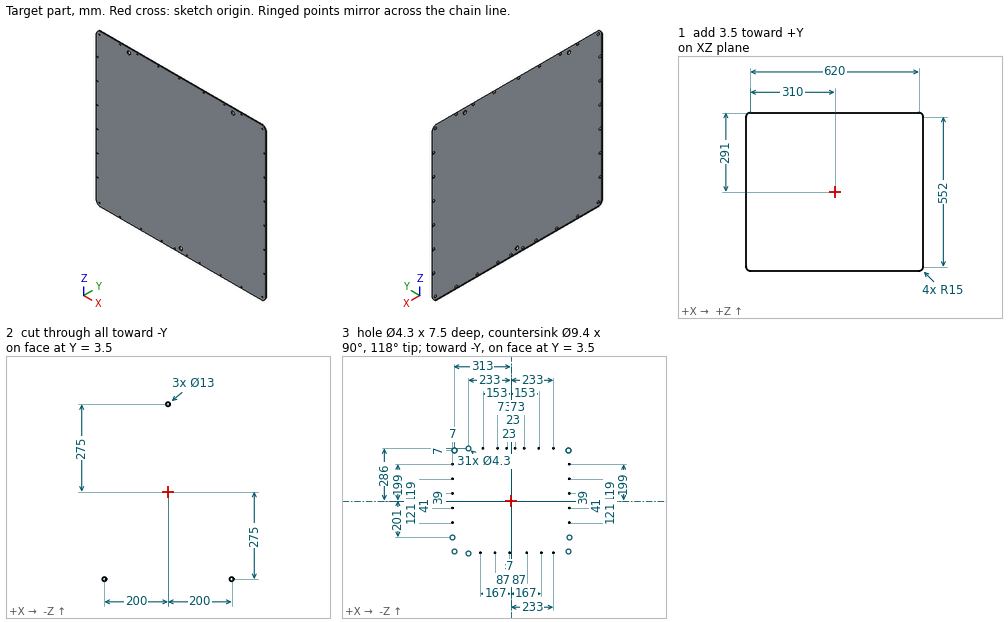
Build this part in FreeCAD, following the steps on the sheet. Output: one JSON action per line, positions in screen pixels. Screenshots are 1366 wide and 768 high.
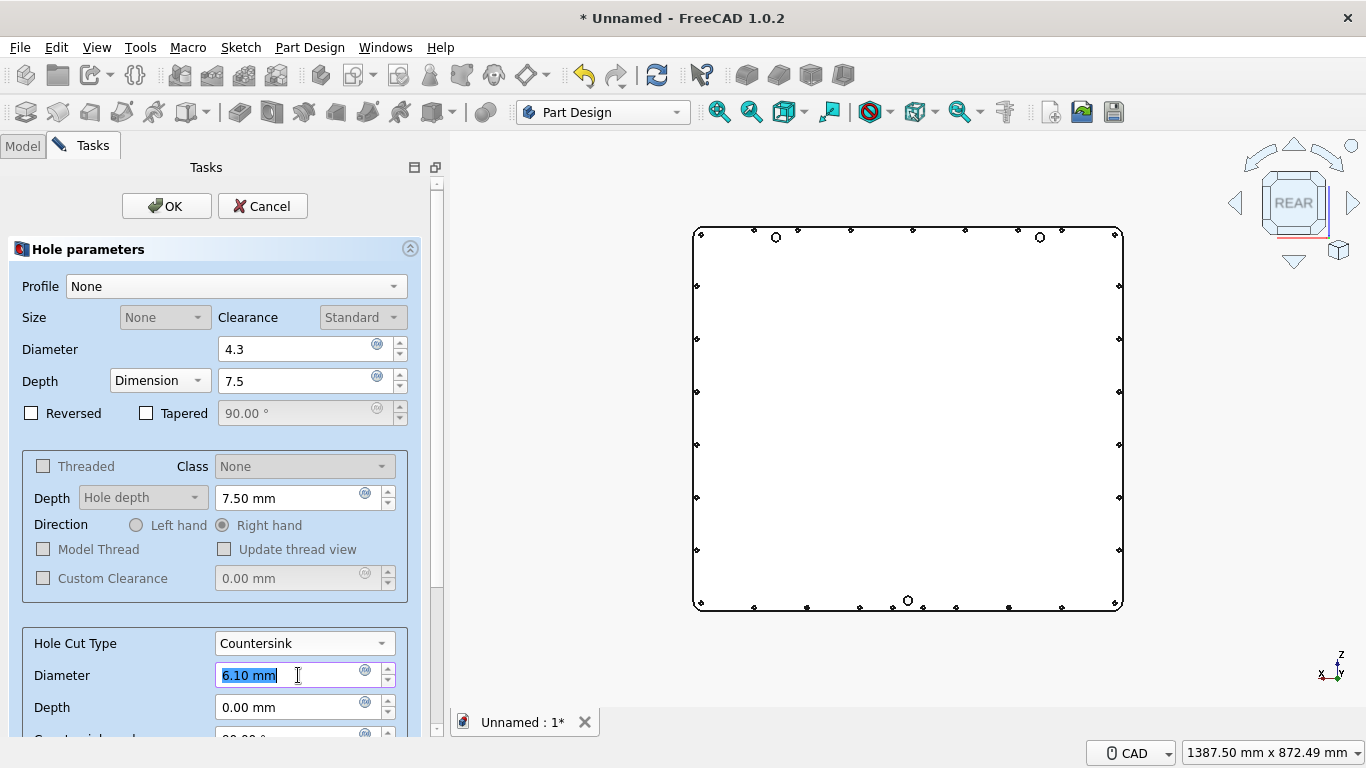
{"action": "type", "text": "9.4"}
{"action": "key", "text": "Tab"}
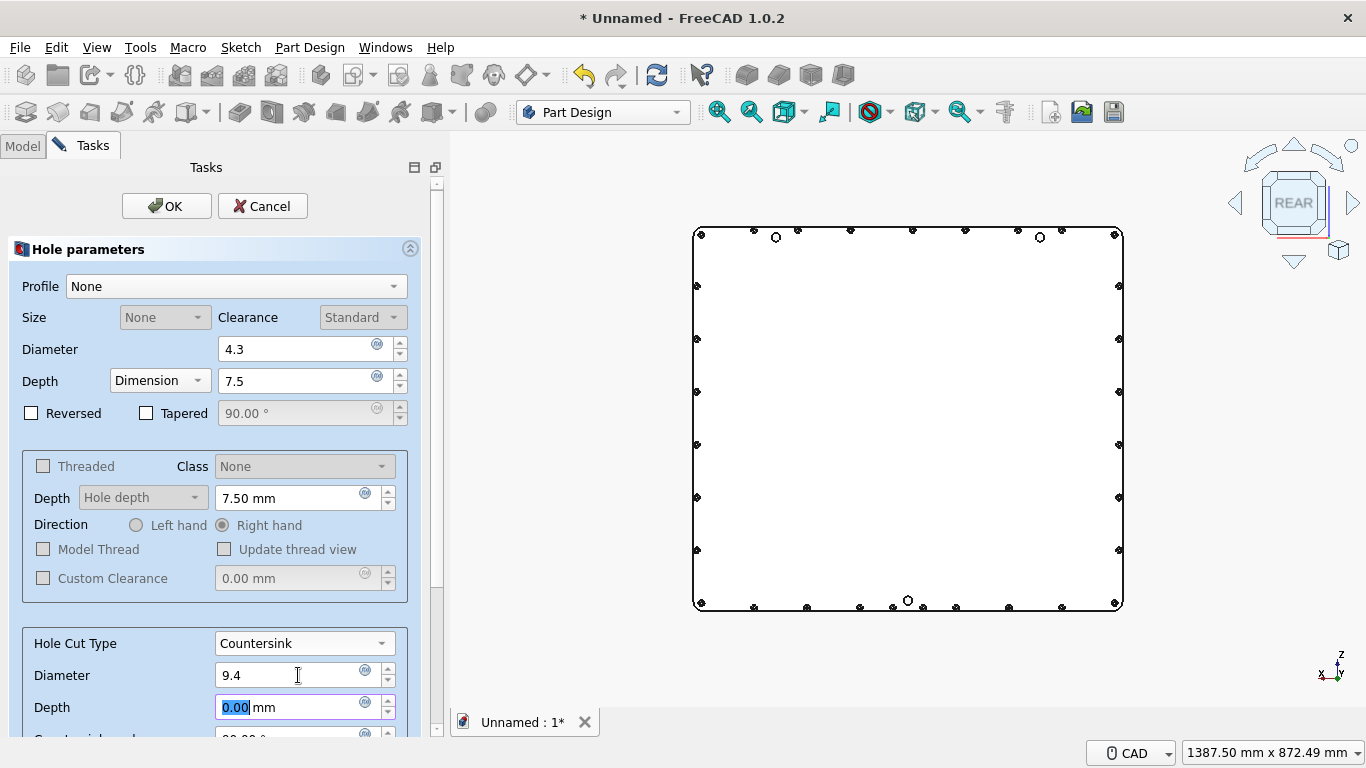
{"action": "left_click", "coordinate": [167, 206]}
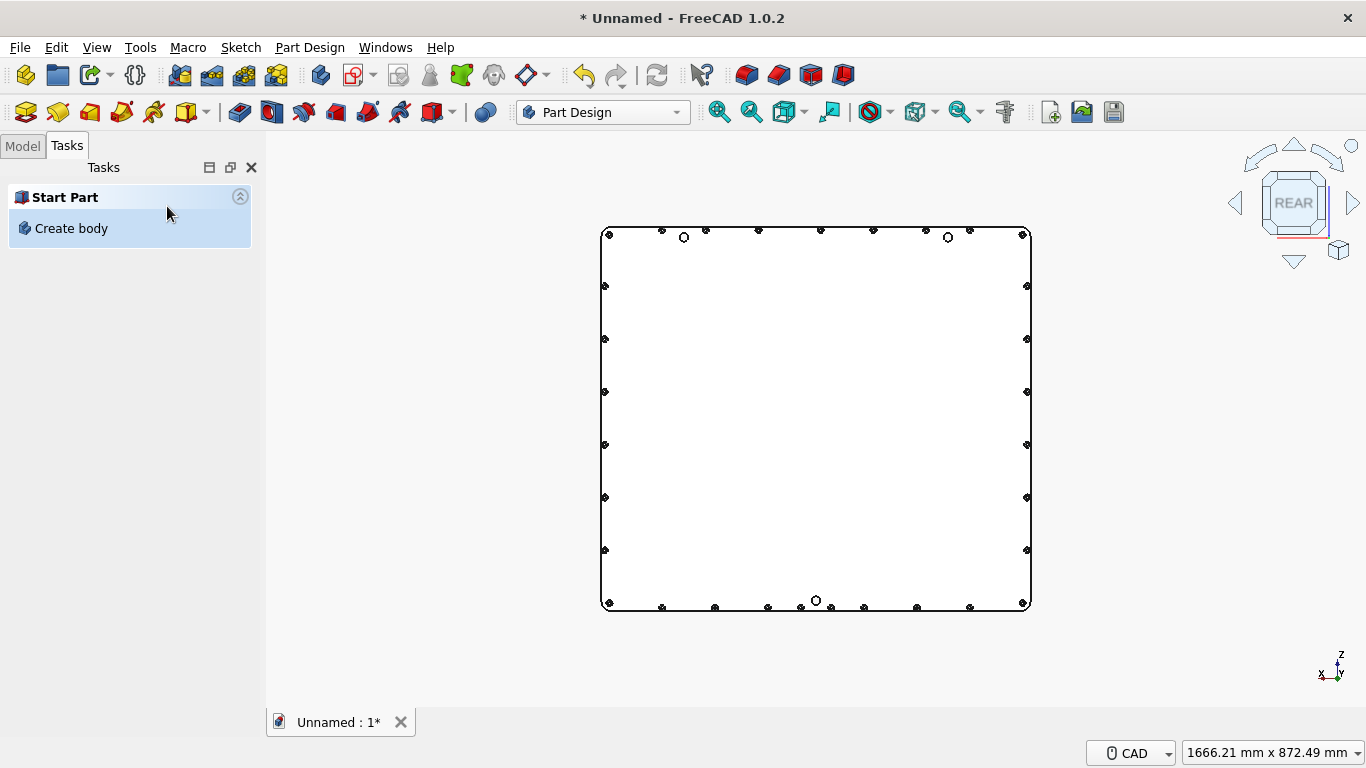
{"action": "key", "text": "0"}